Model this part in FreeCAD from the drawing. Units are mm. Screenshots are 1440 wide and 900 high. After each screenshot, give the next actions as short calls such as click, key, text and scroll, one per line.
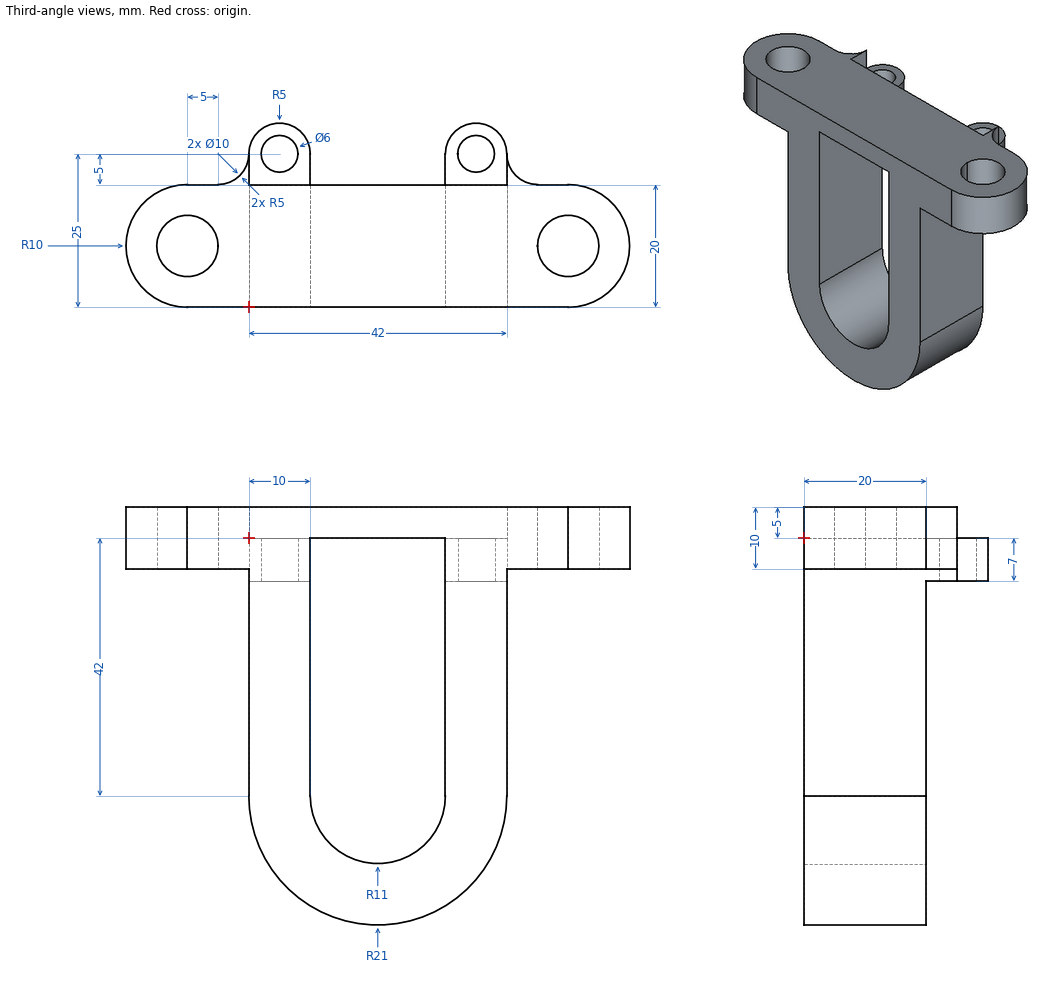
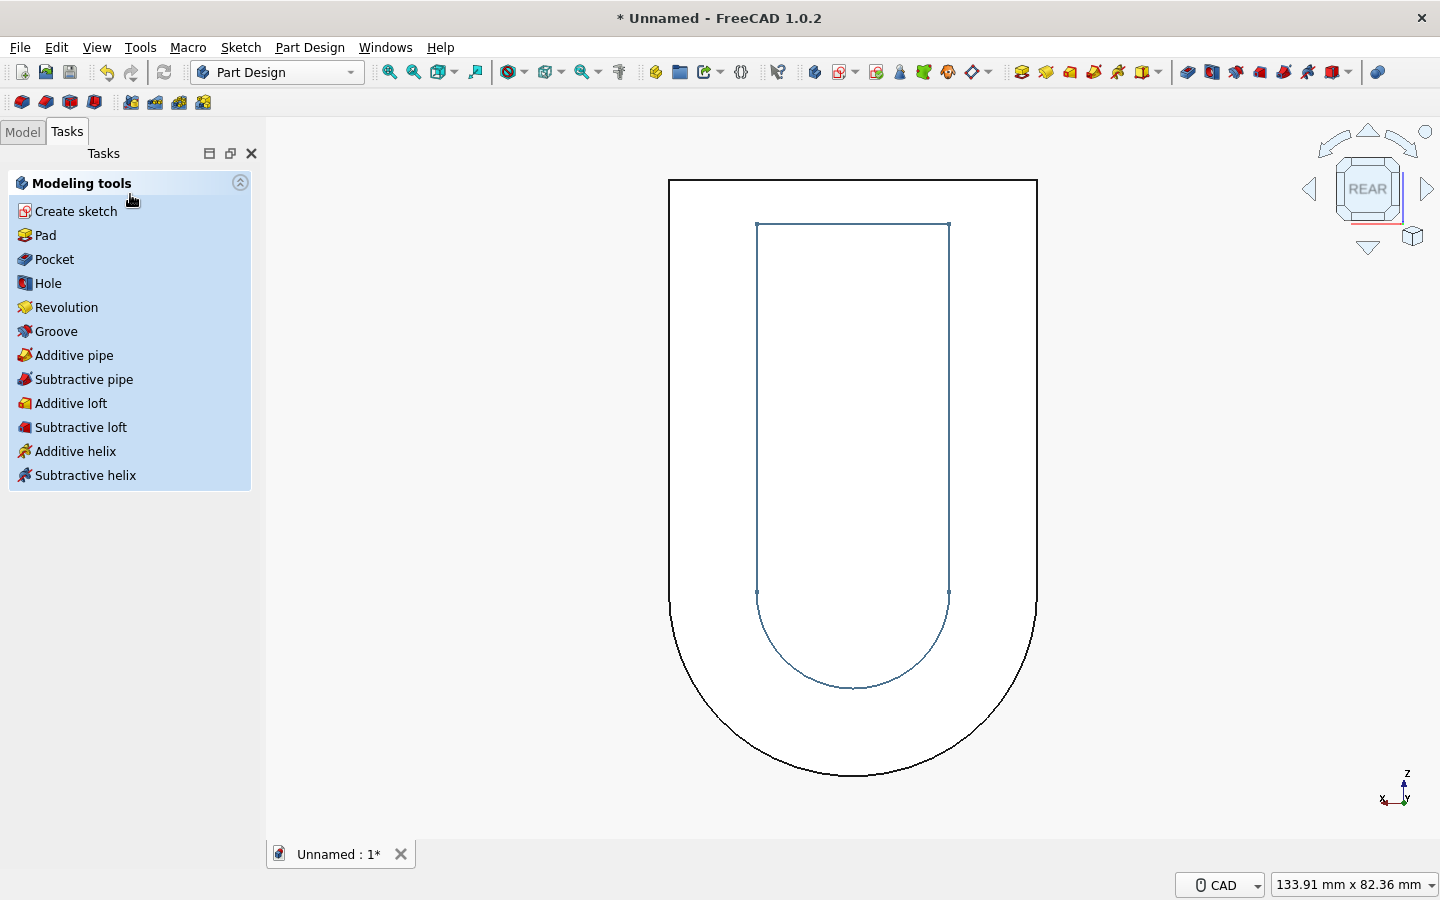
click(1188, 72)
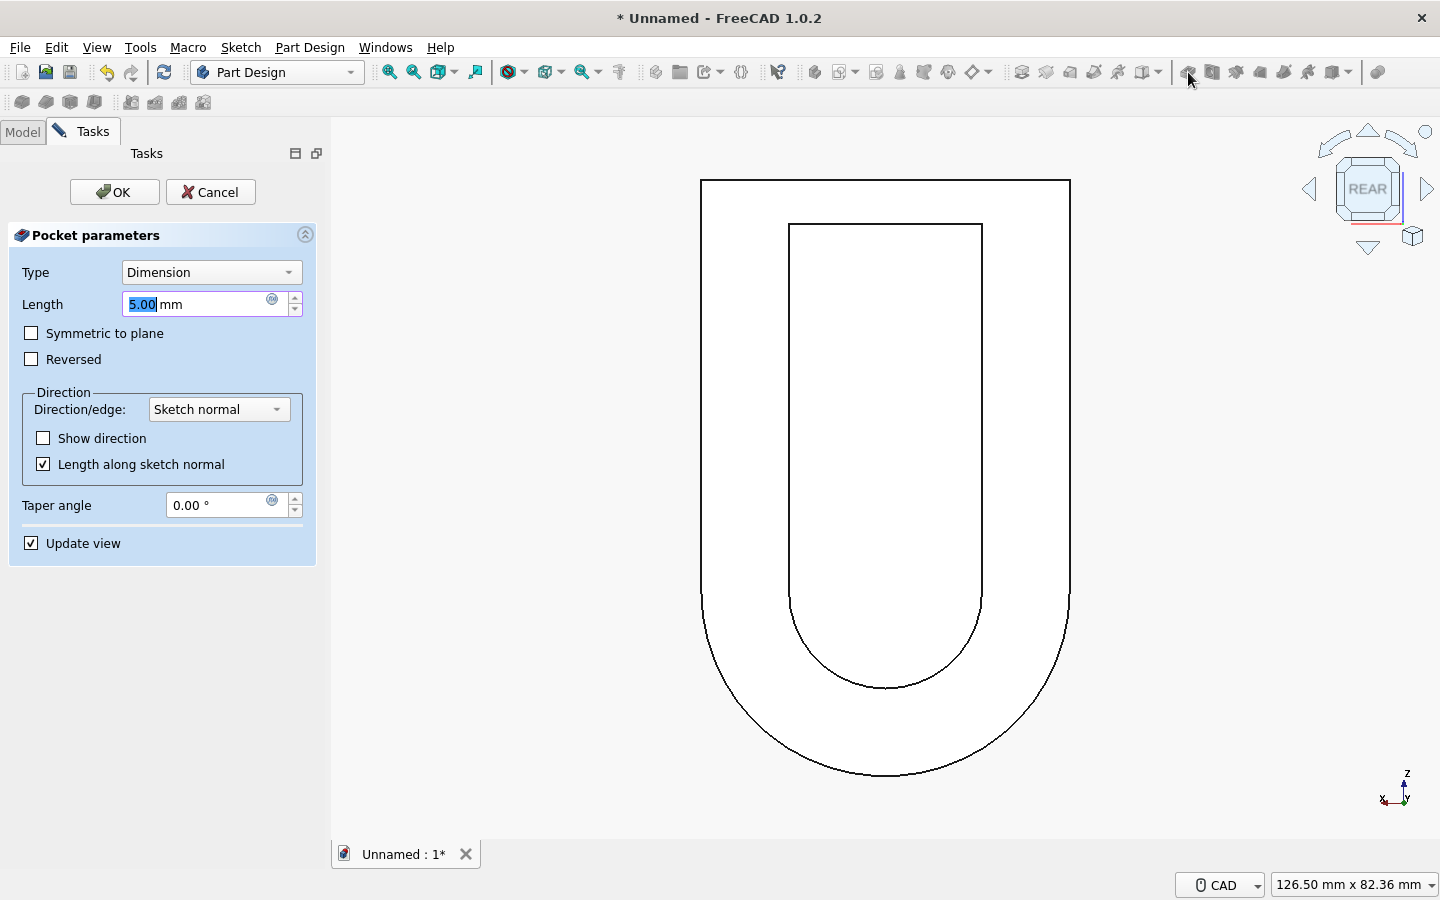
click(212, 272)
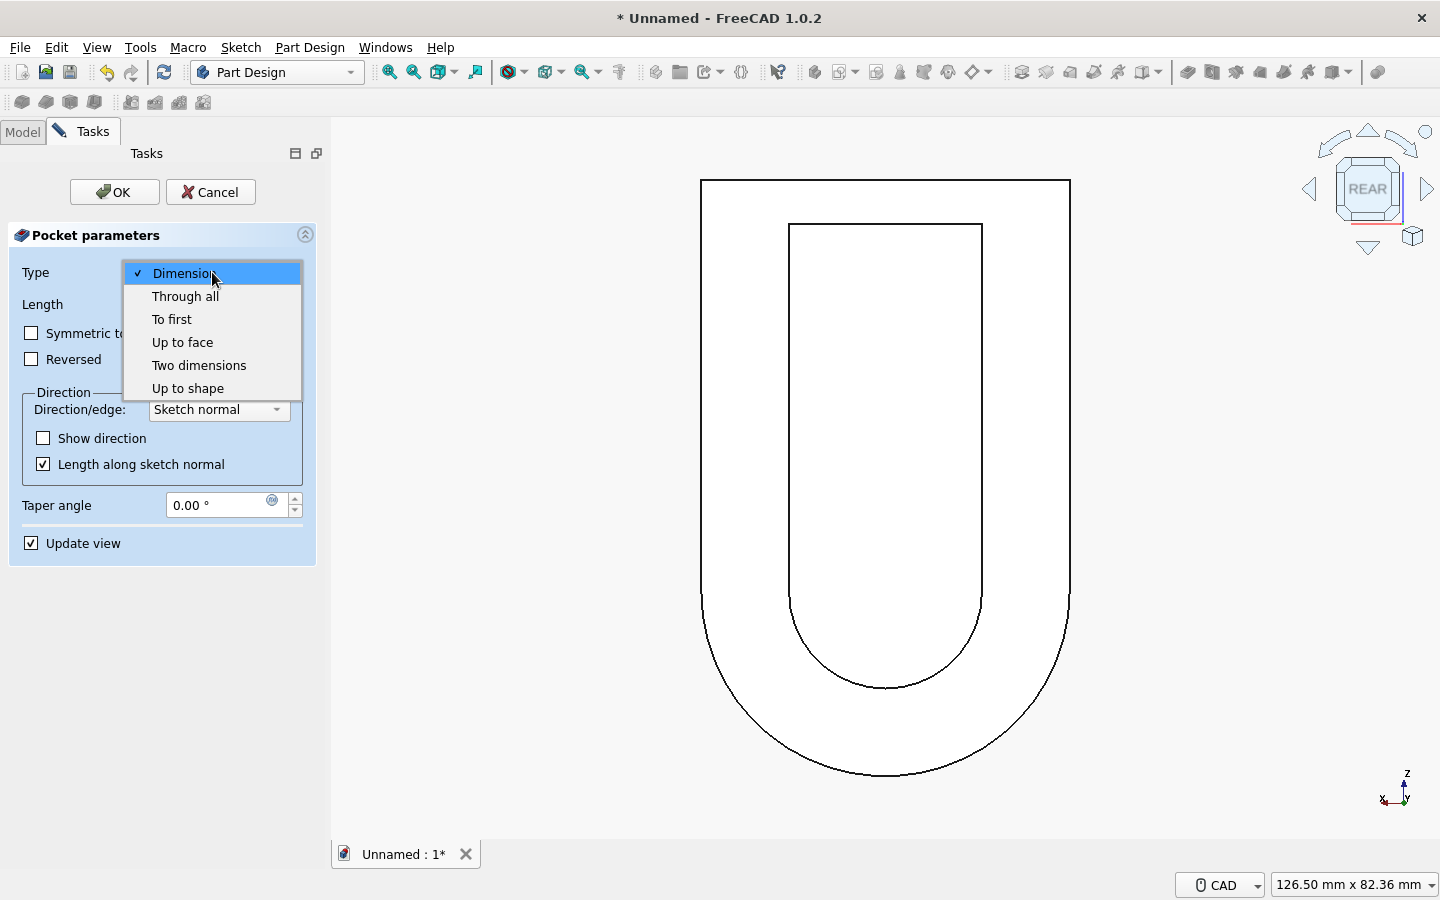
click(212, 296)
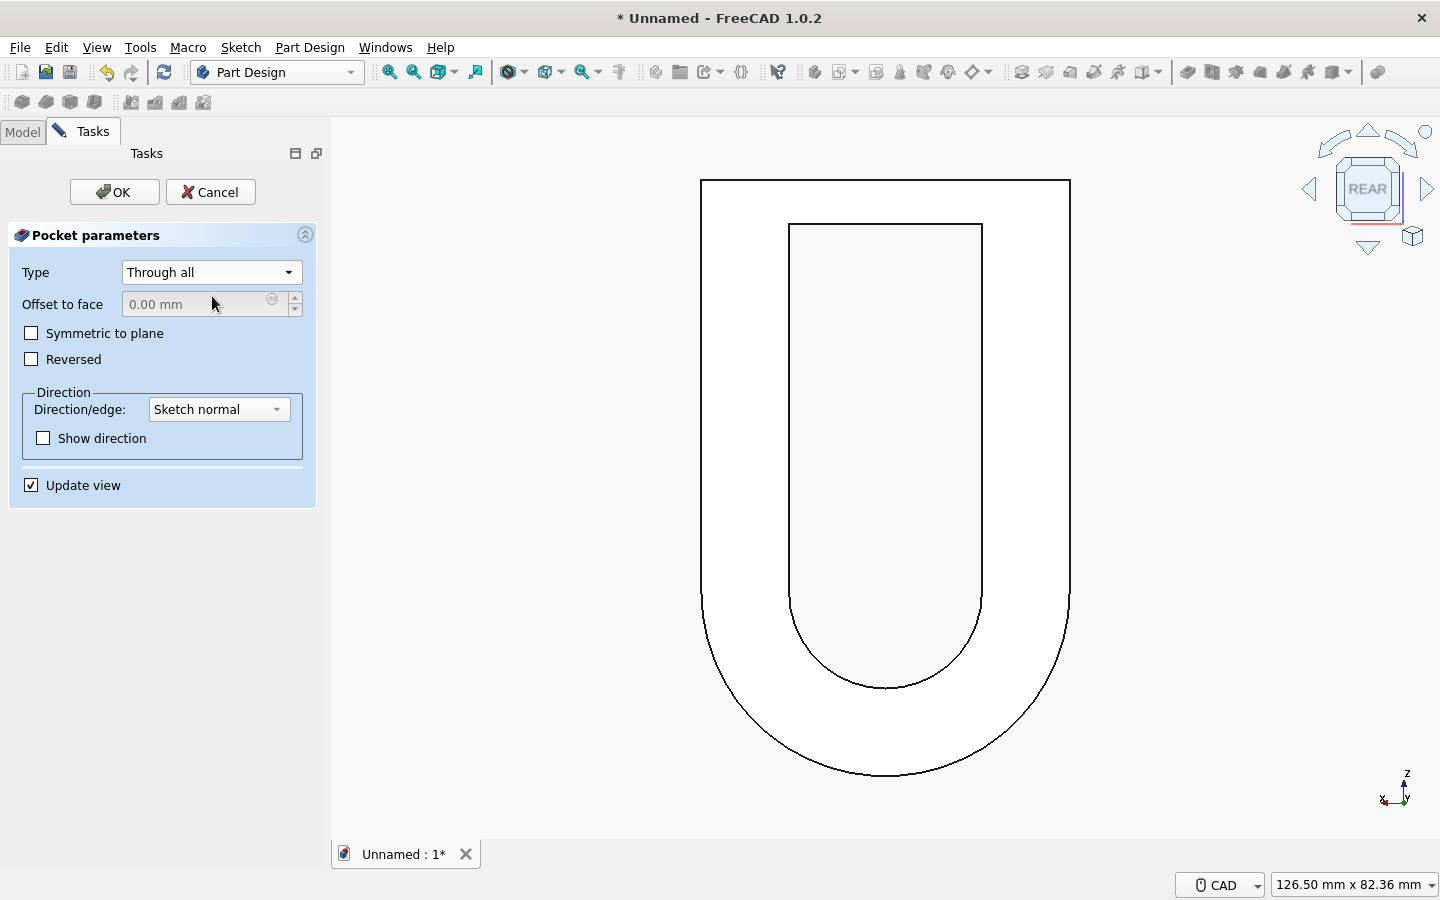
click(115, 192)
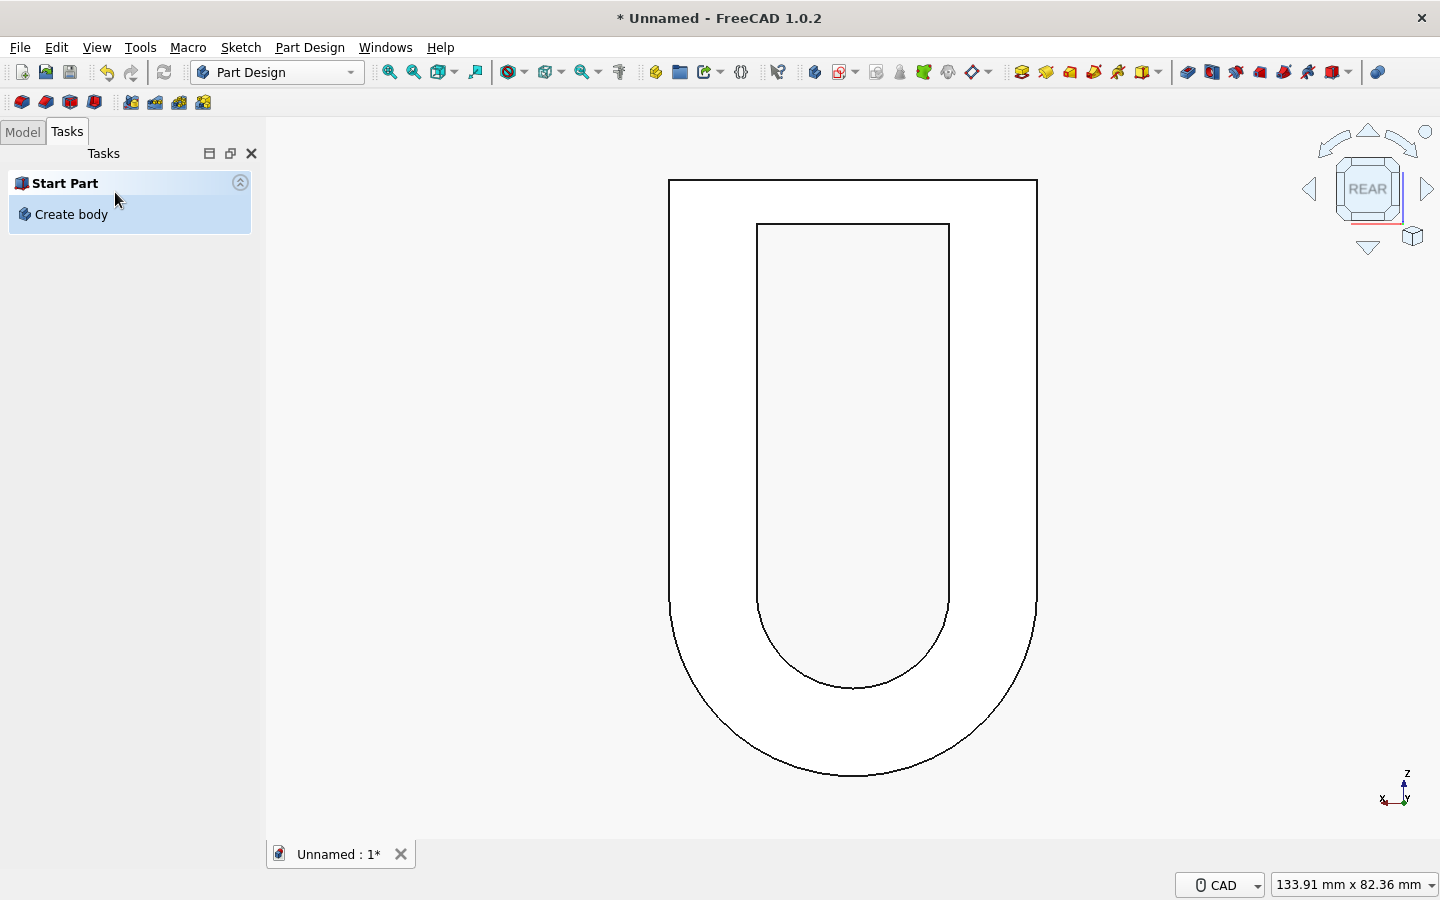
click(840, 72)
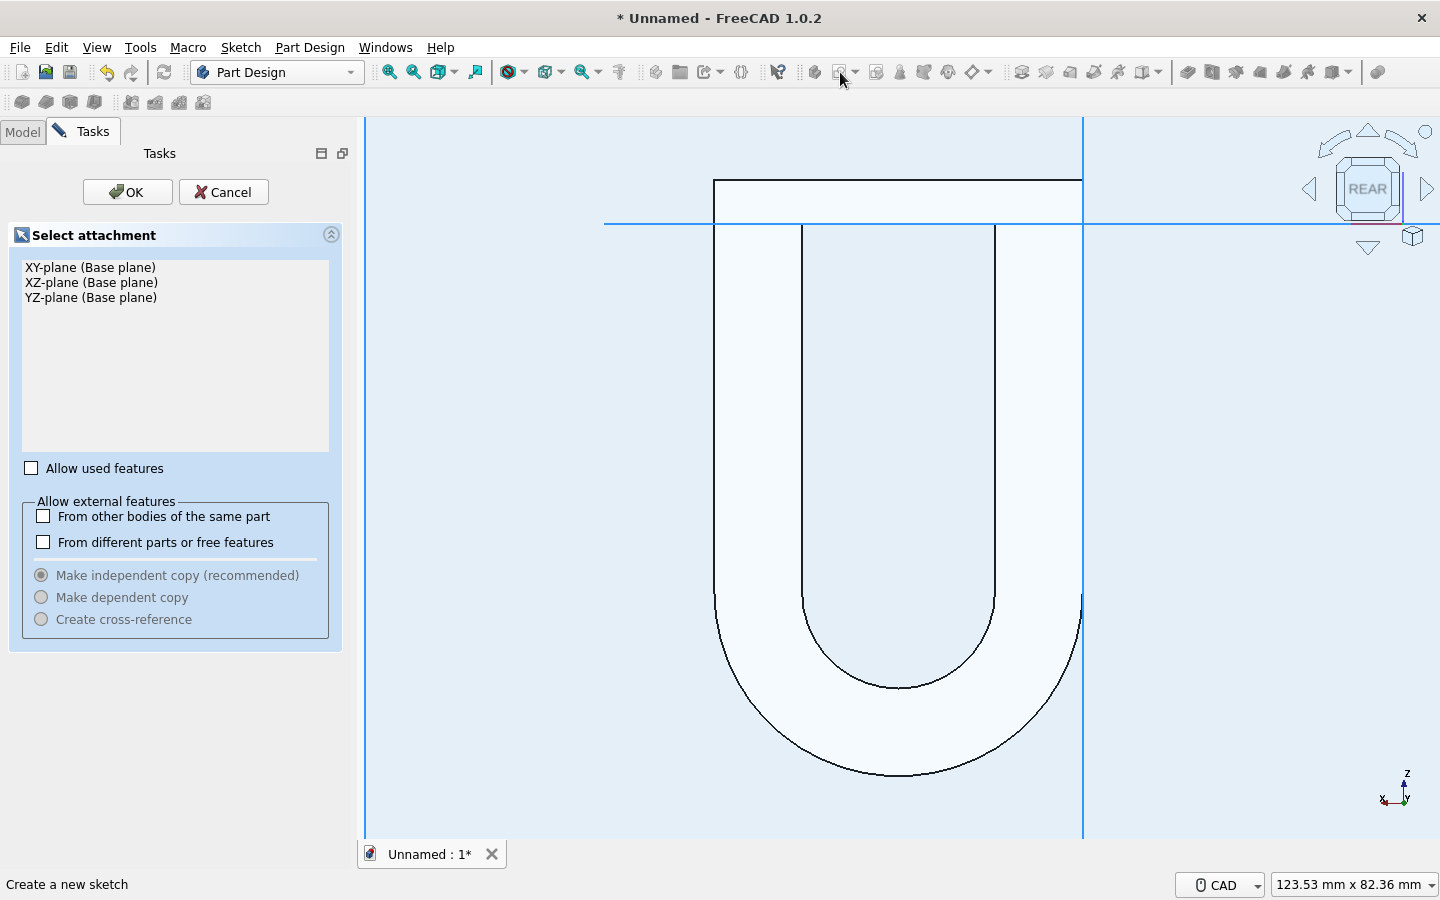
click(82, 268)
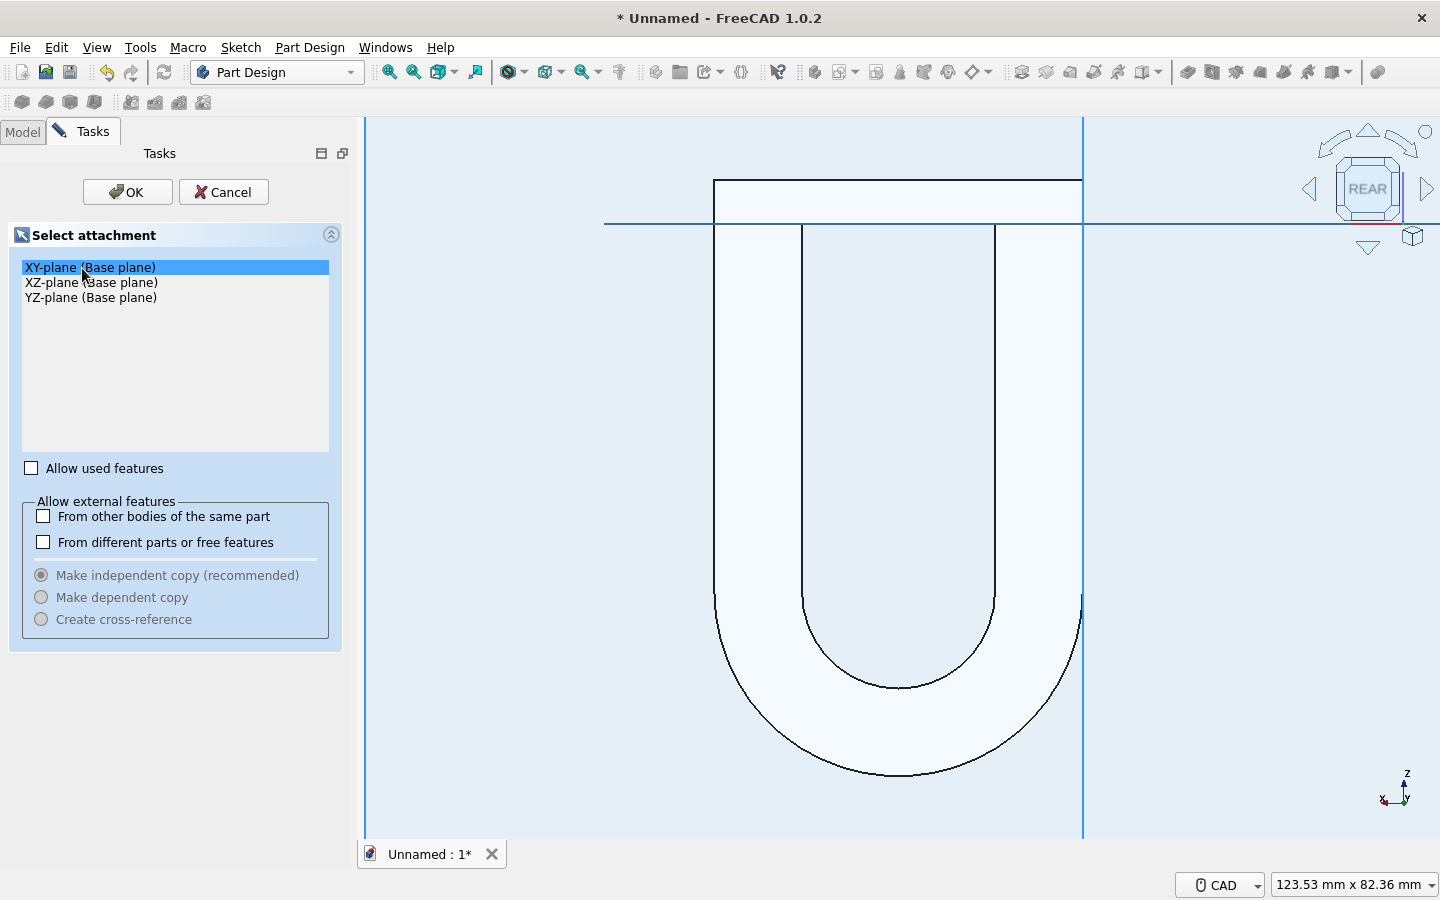
click(128, 192)